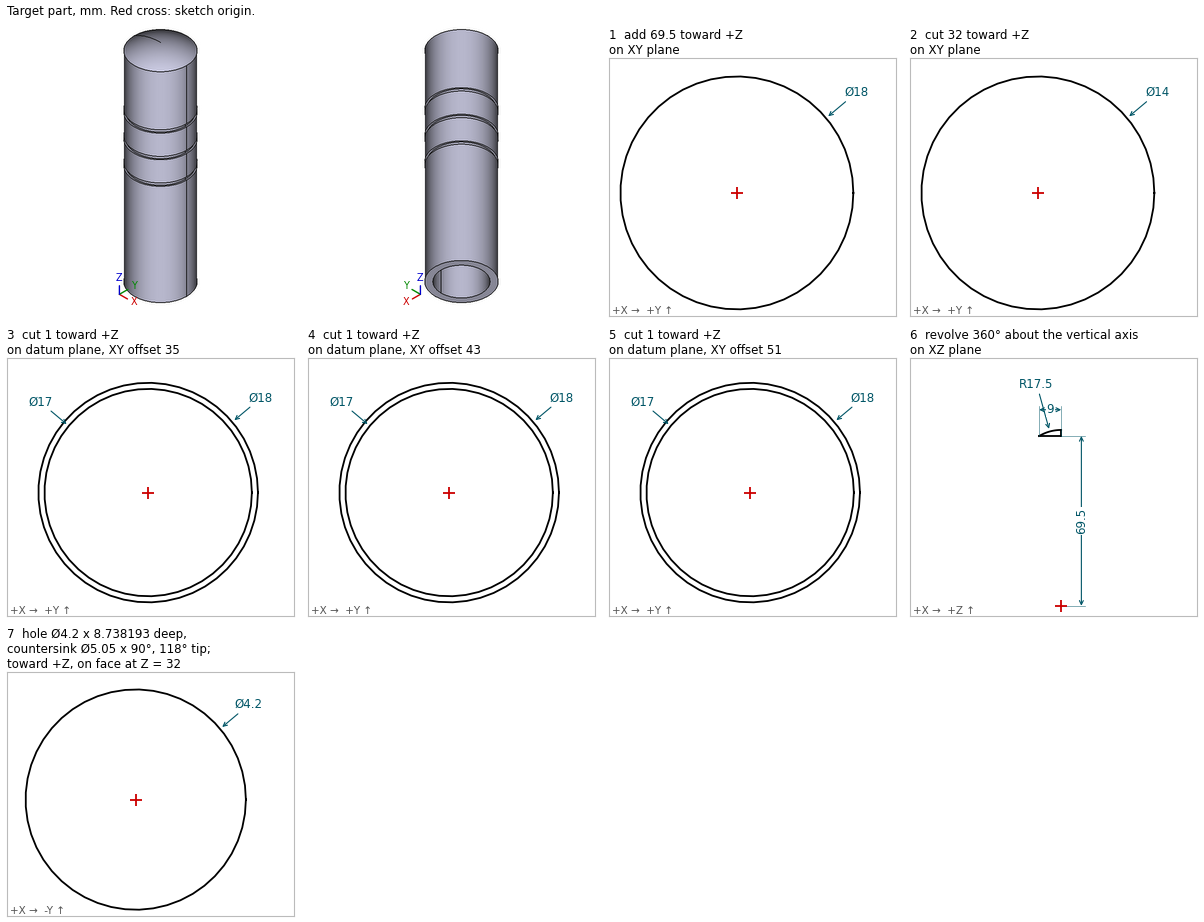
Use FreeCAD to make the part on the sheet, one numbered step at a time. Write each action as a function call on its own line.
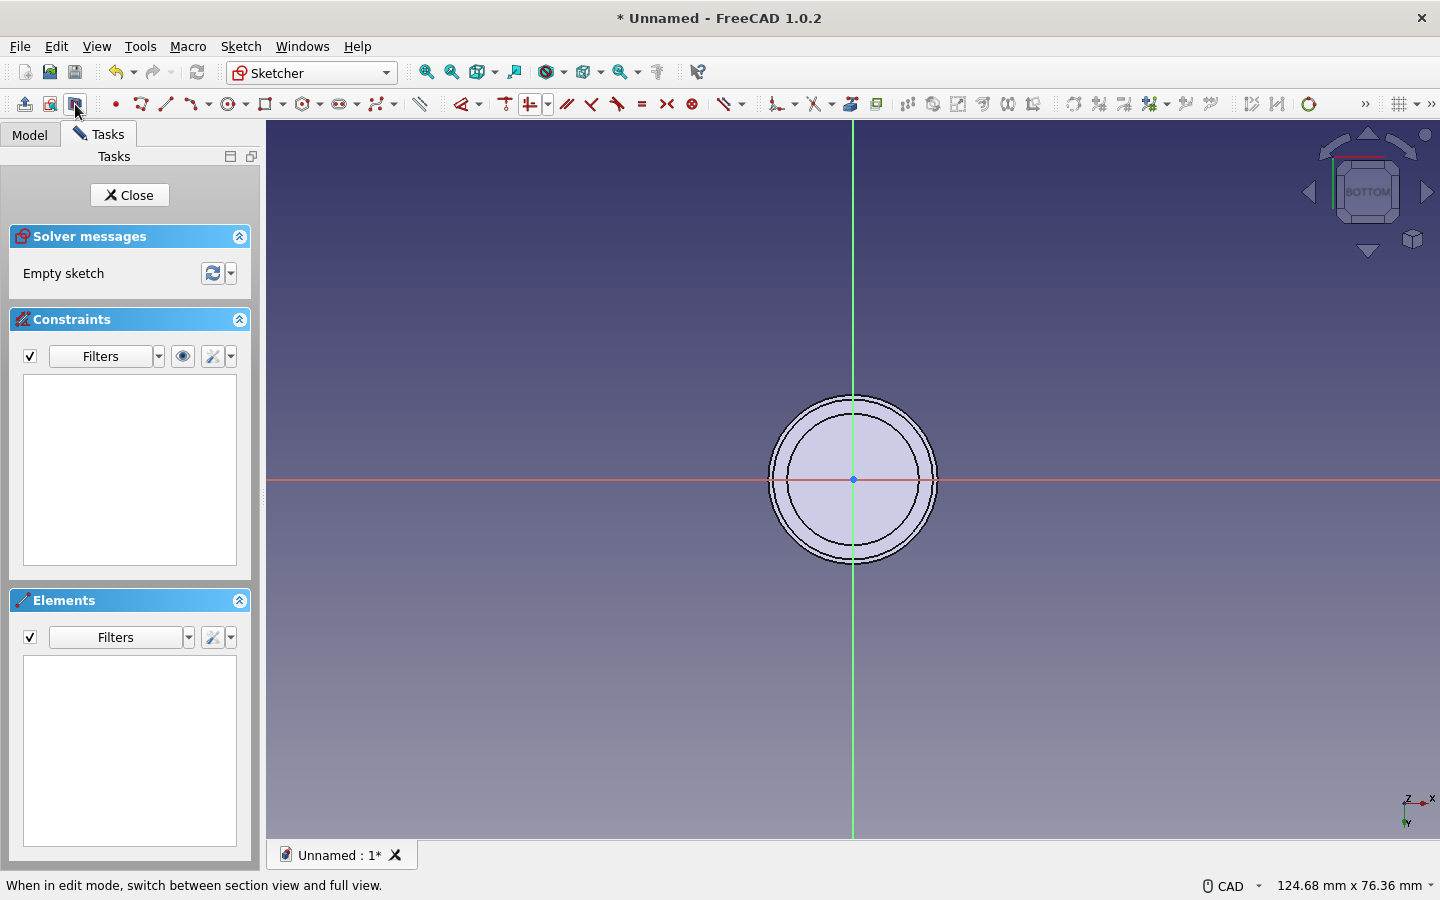
scroll(860, 480, up, 12)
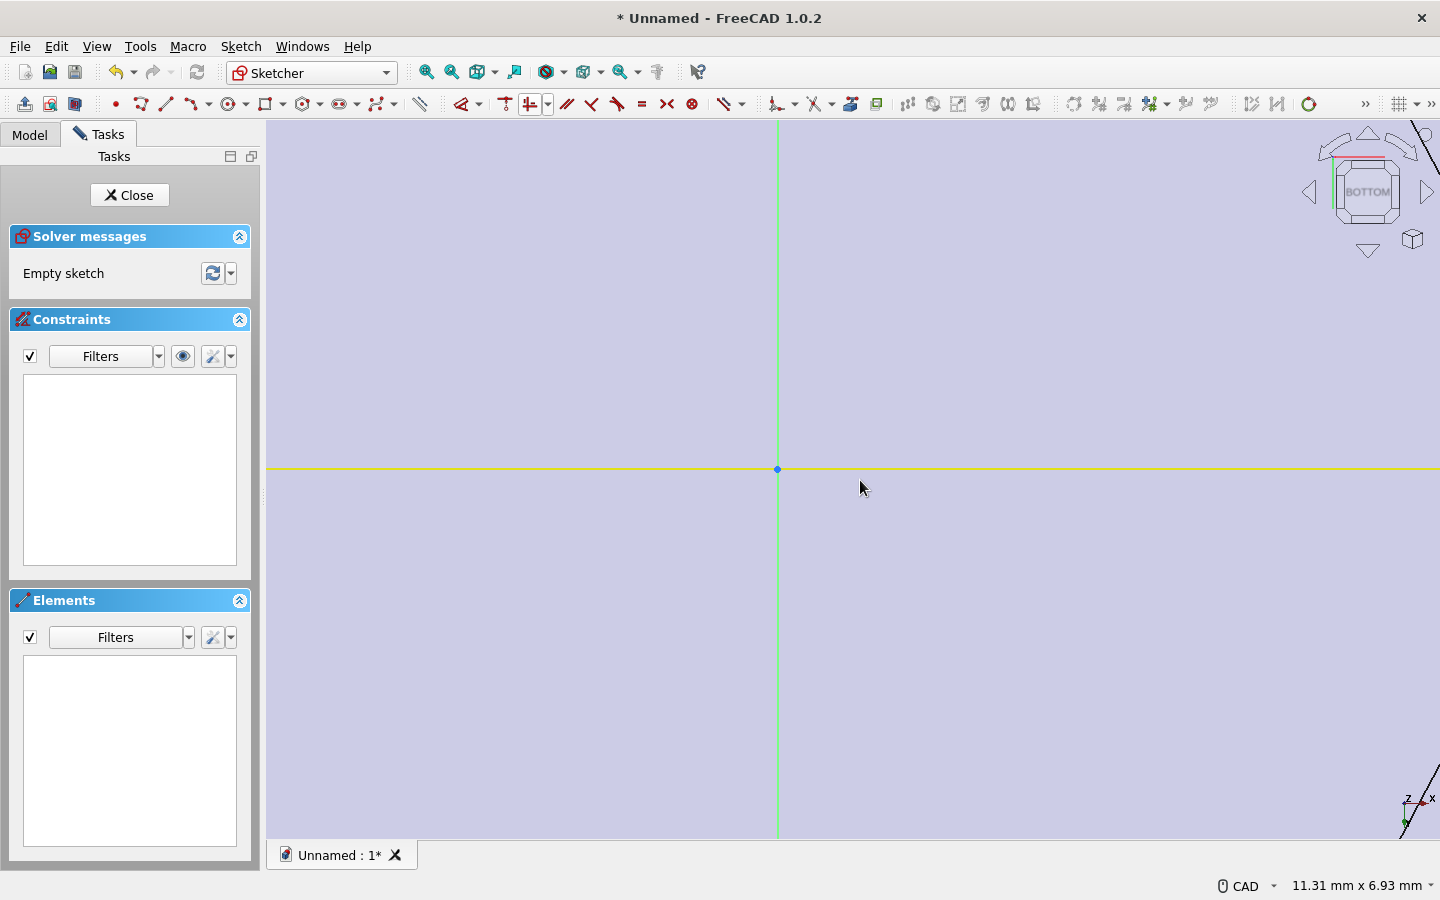
key(g)
key(c)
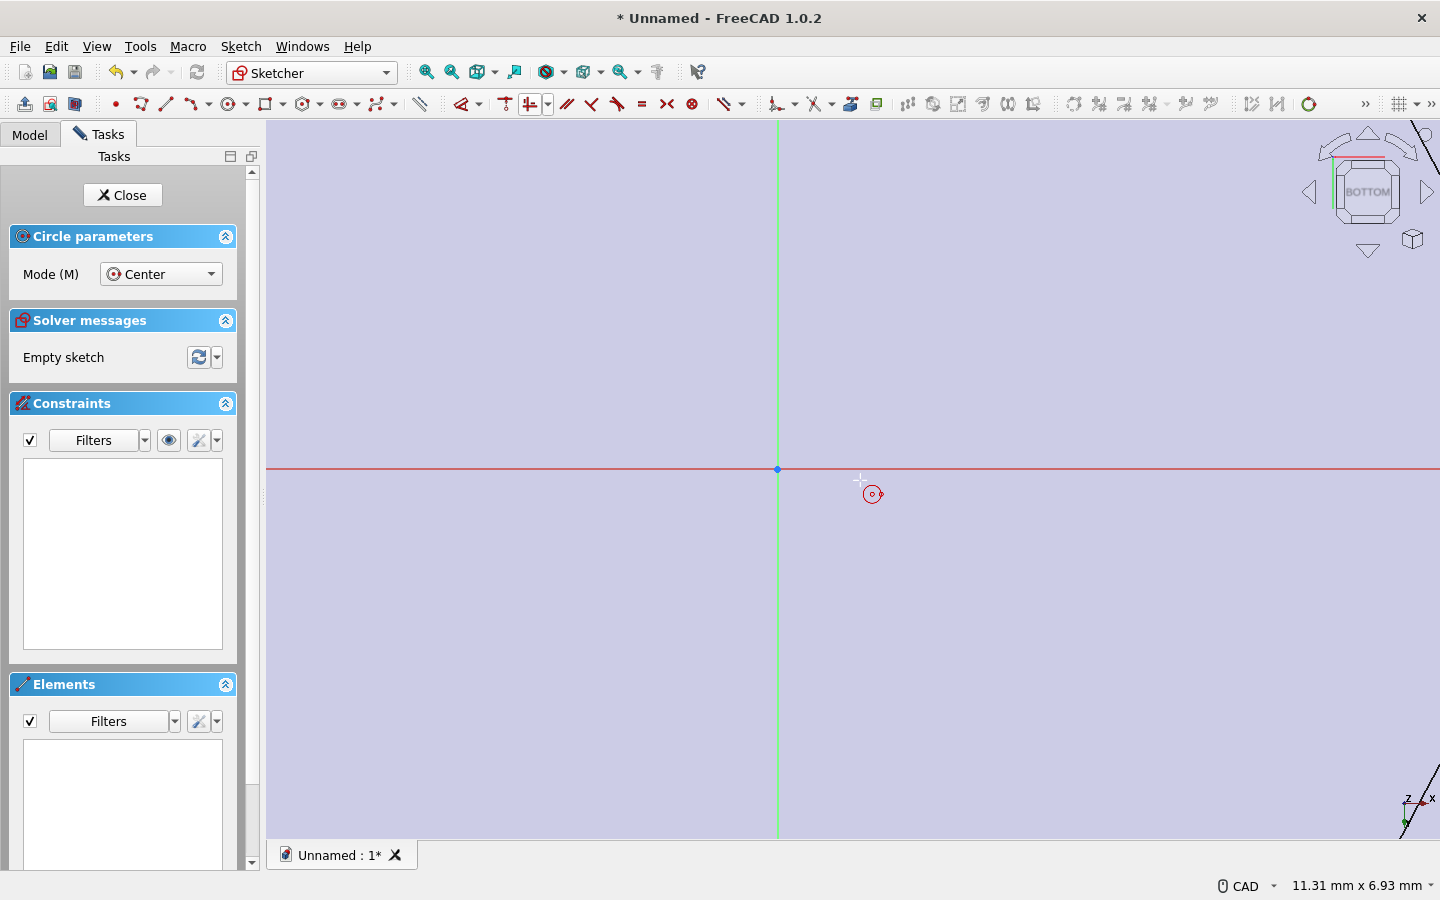
click(778, 469)
click(932, 315)
key(Escape)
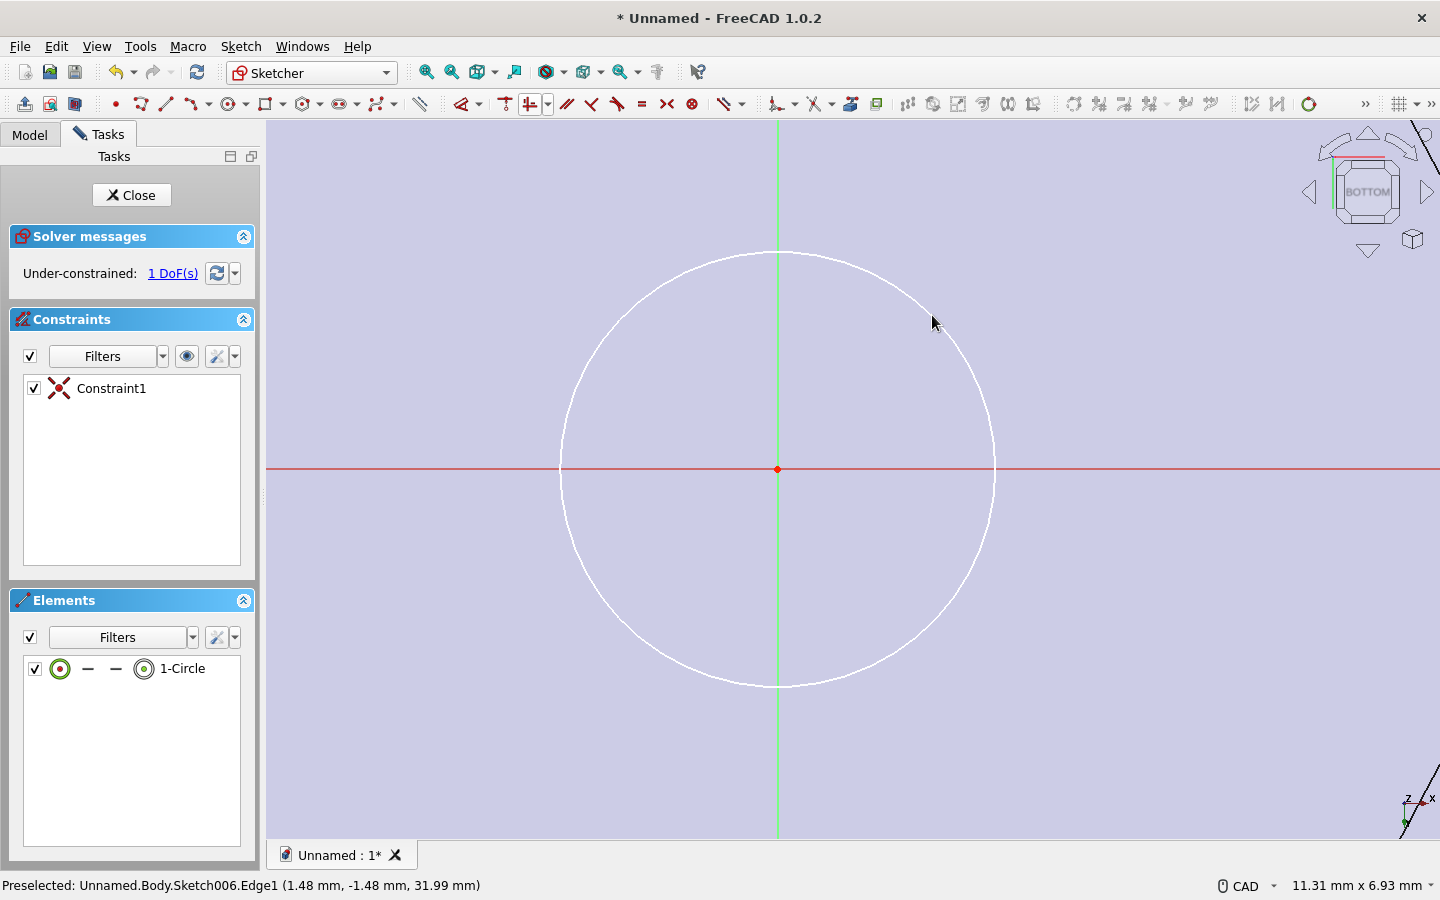
key(d)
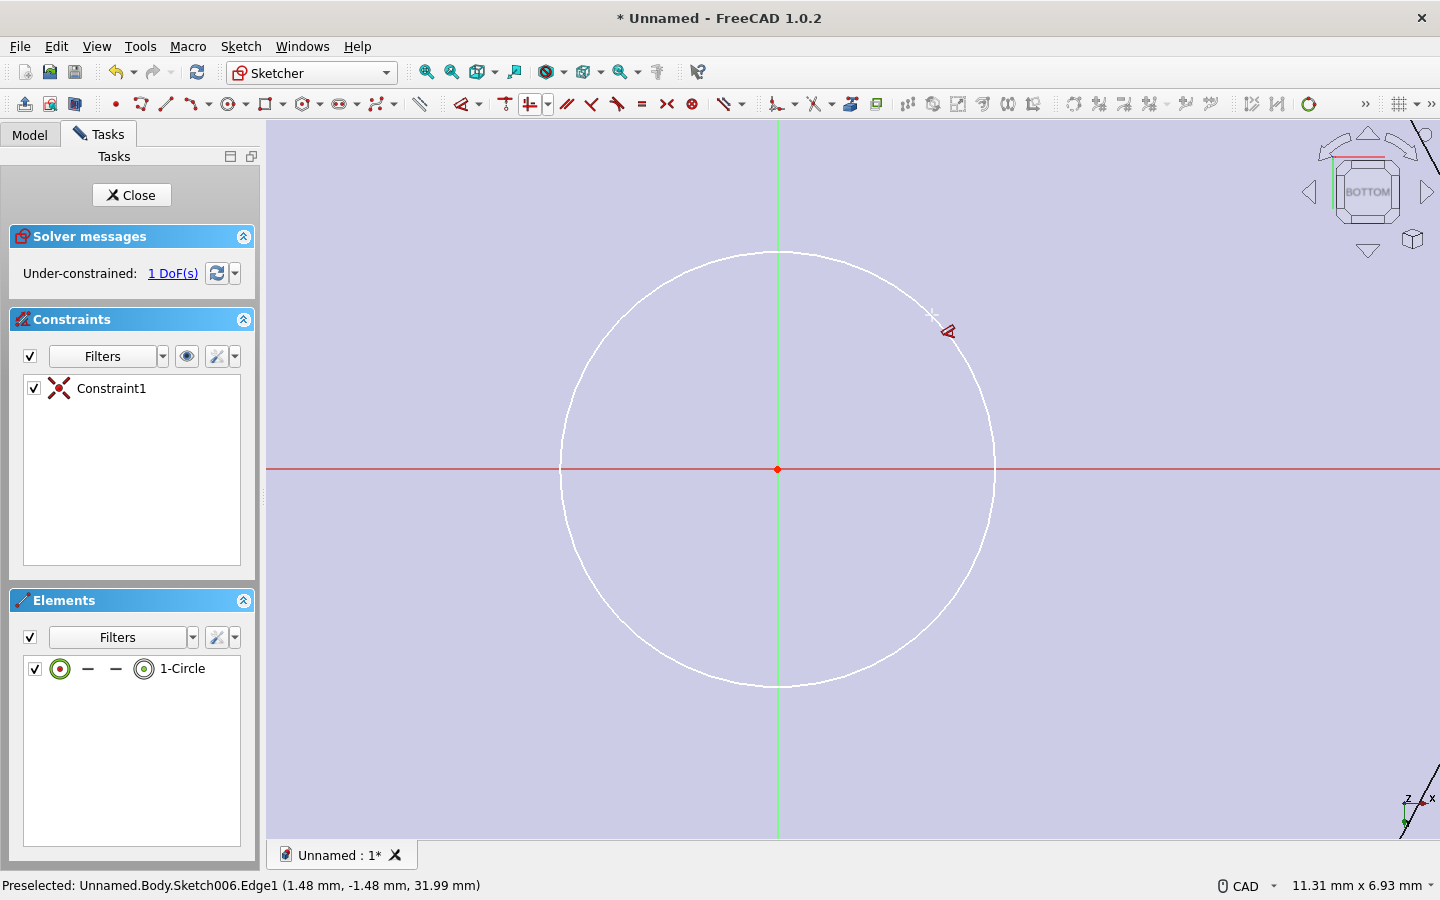
click(931, 315)
click(954, 292)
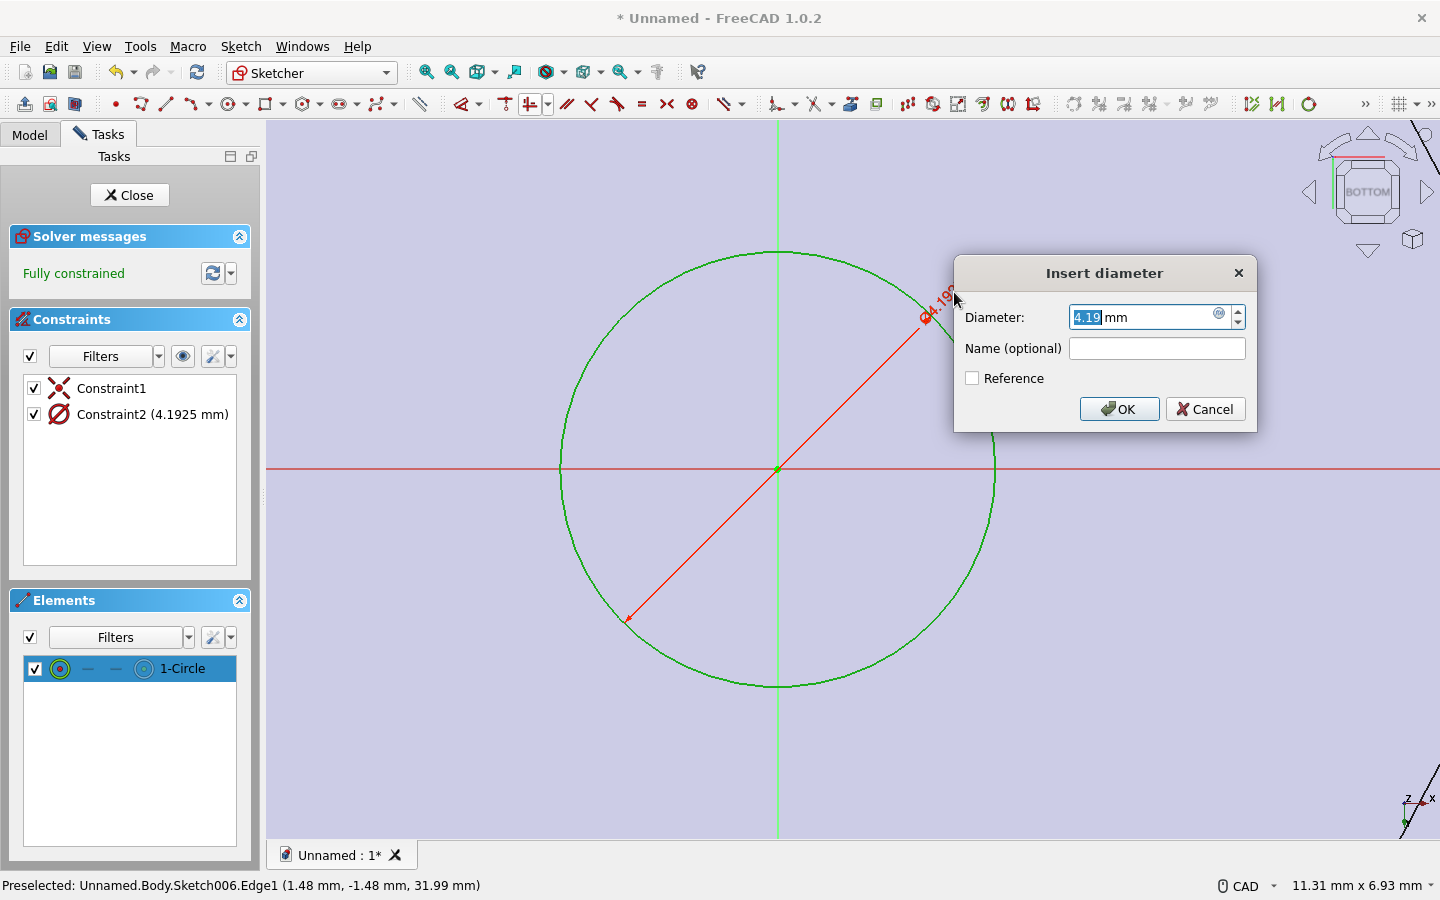
text(4.2)
key(Return)
key(Escape)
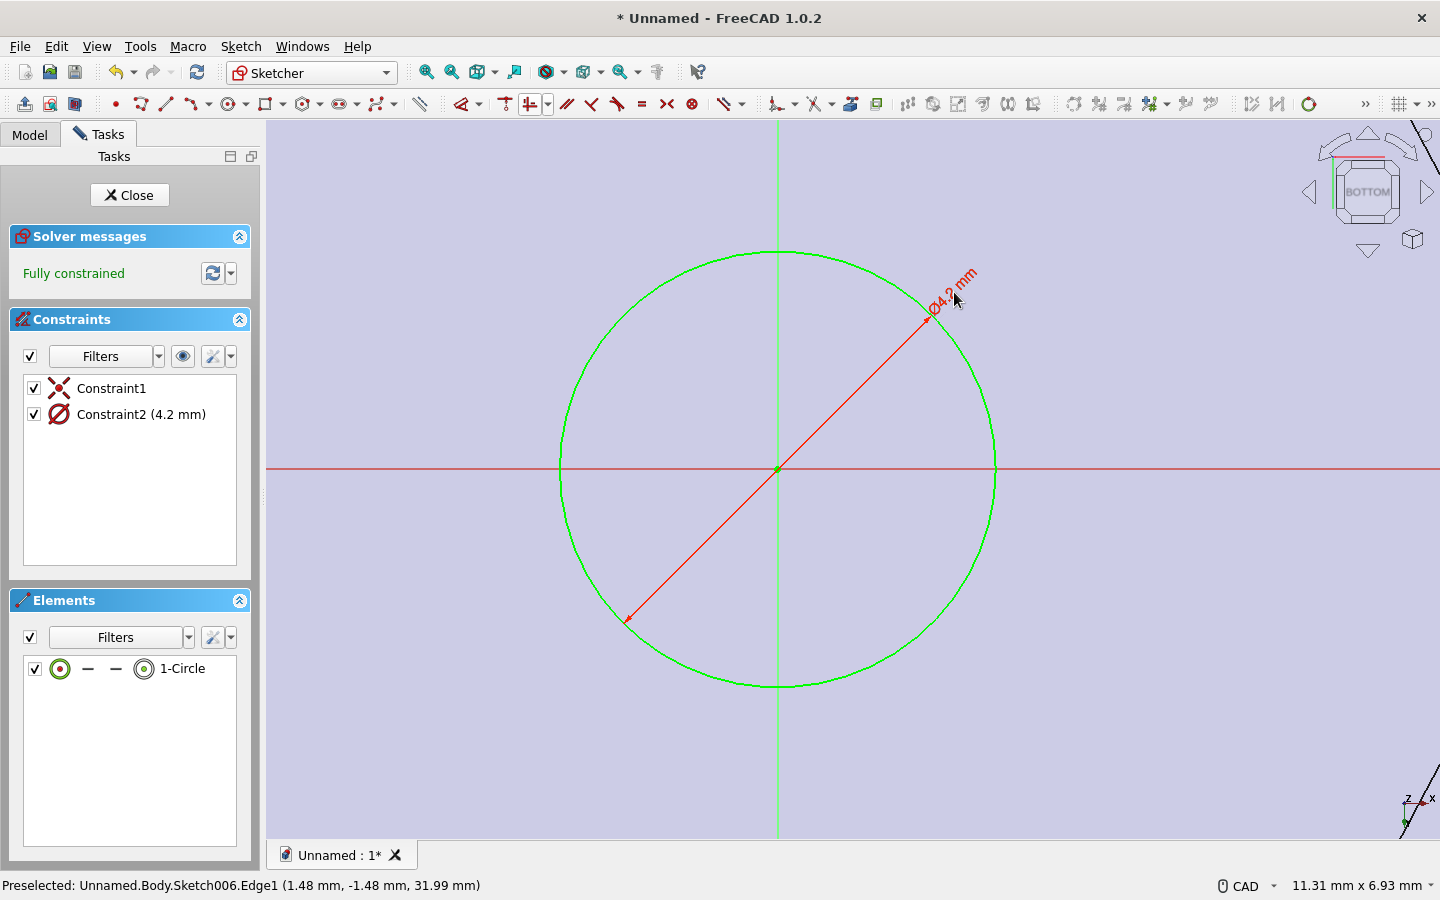
click(130, 195)